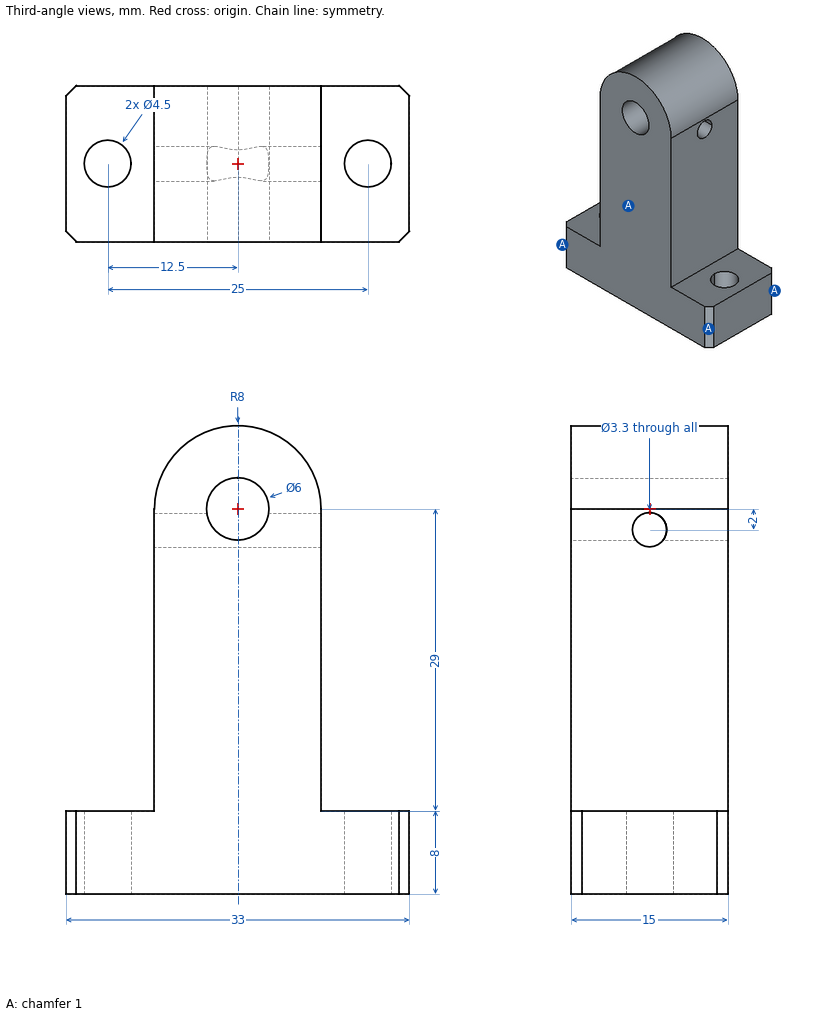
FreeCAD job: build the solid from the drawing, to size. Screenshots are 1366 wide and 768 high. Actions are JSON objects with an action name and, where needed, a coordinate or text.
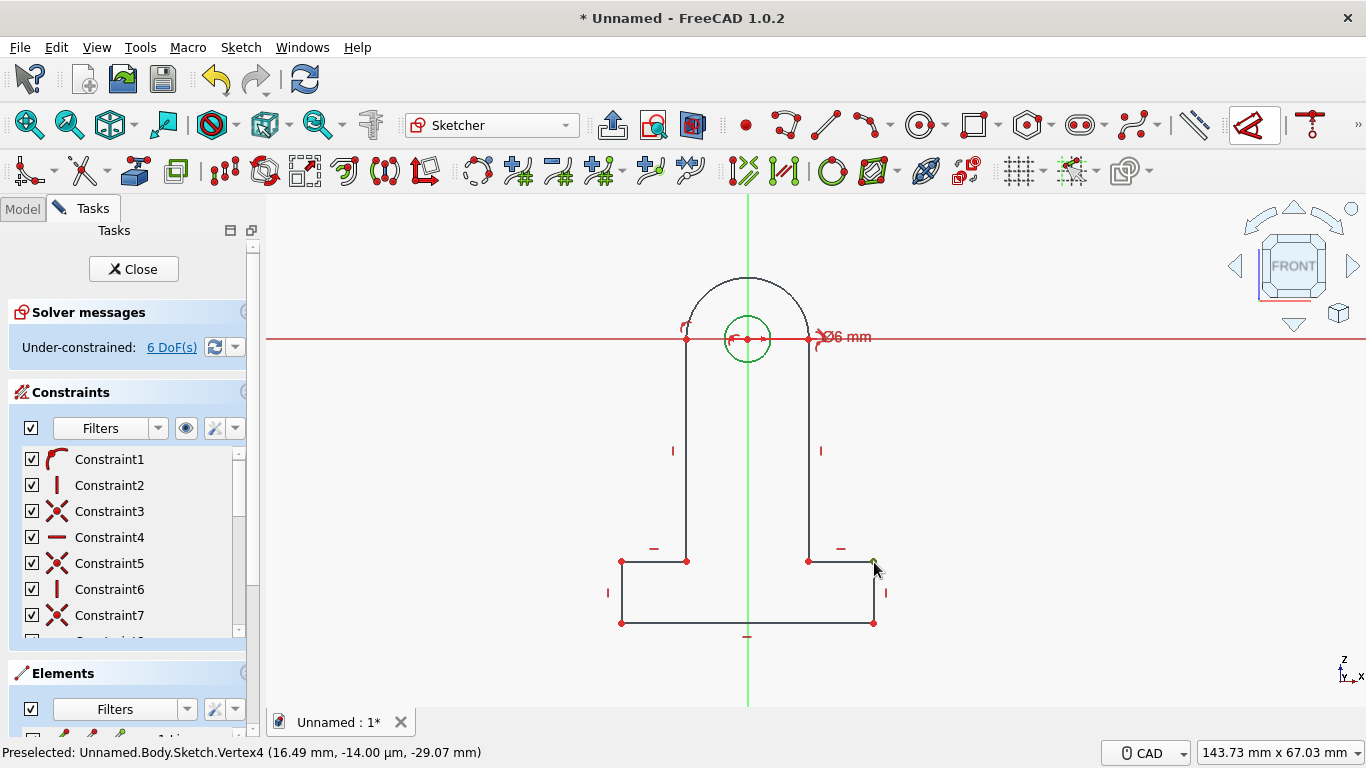
{"action": "left_click", "coordinate": [622, 562]}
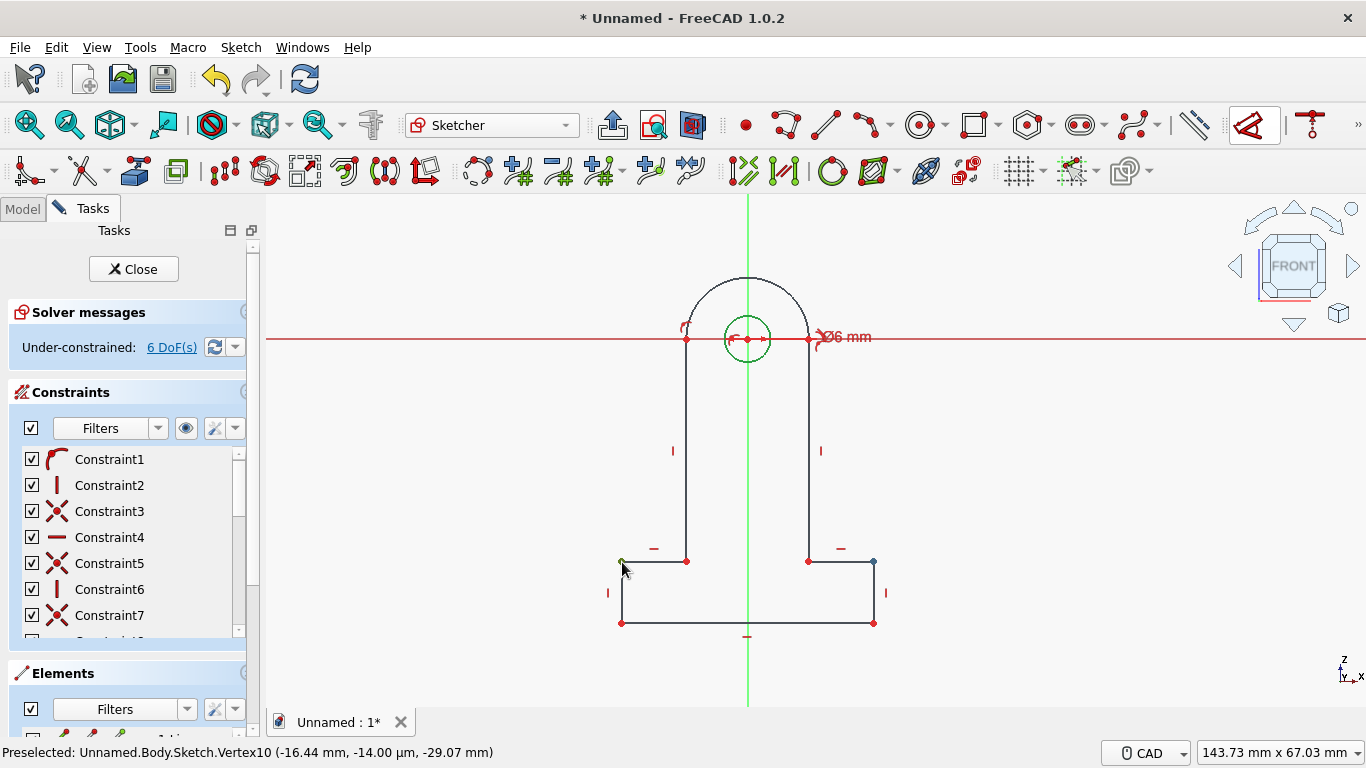
{"action": "left_click", "coordinate": [748, 581]}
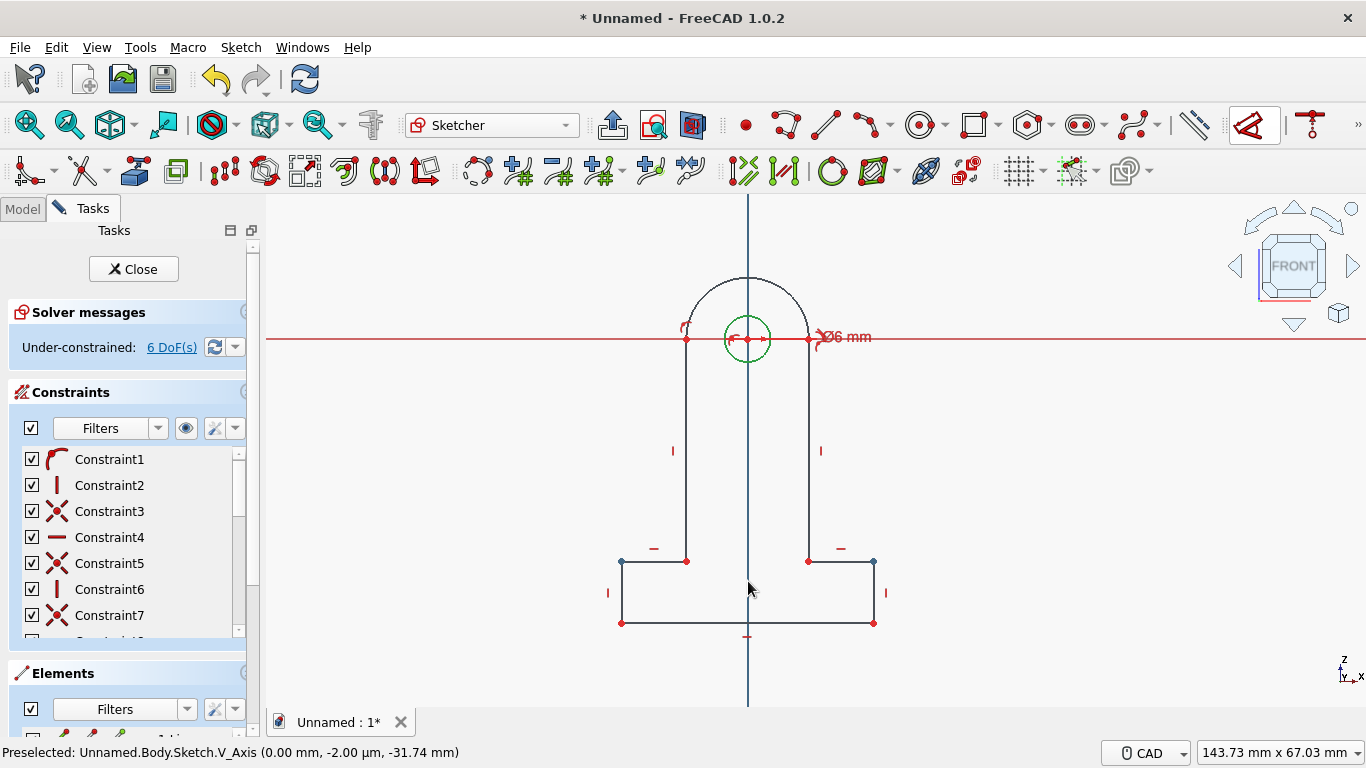
{"action": "key", "text": "s"}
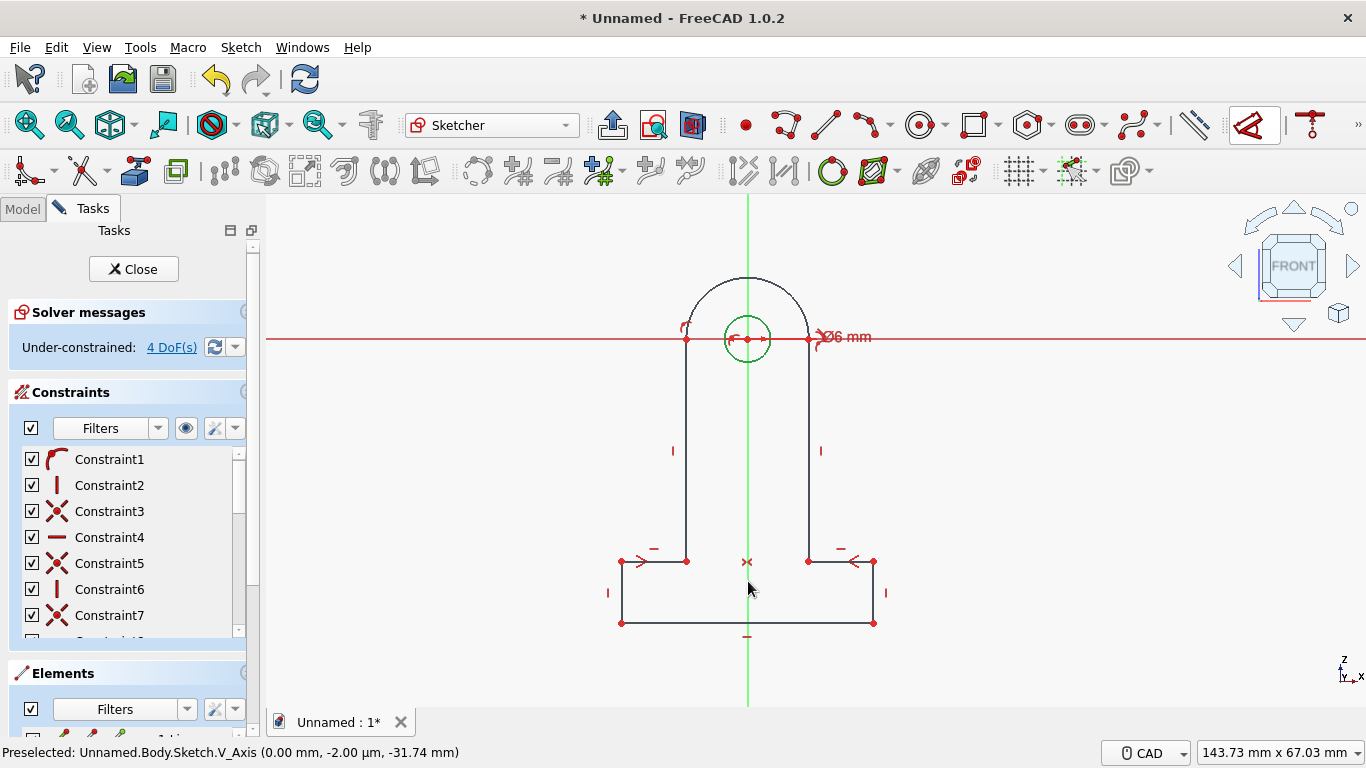
{"action": "key", "text": "d"}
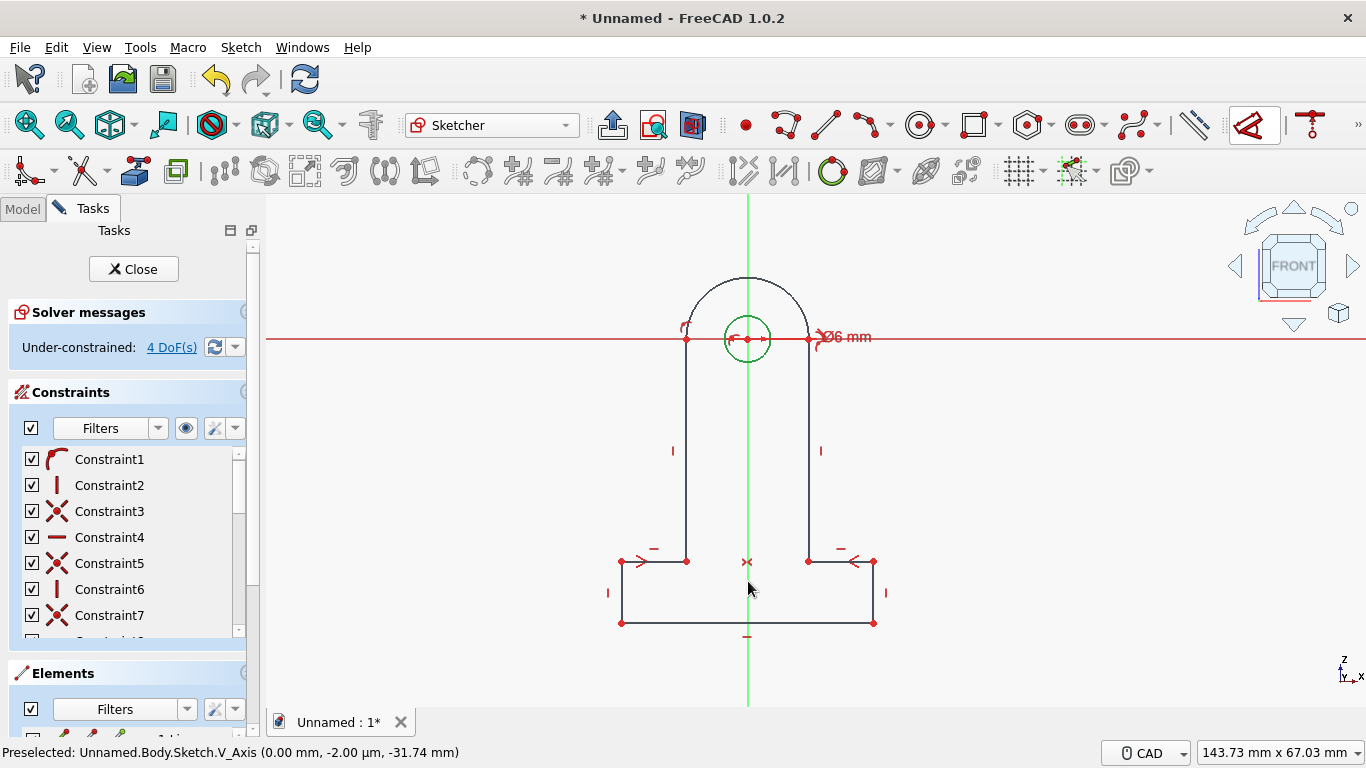
{"action": "left_click", "coordinate": [784, 290]}
{"action": "left_click", "coordinate": [803, 264]}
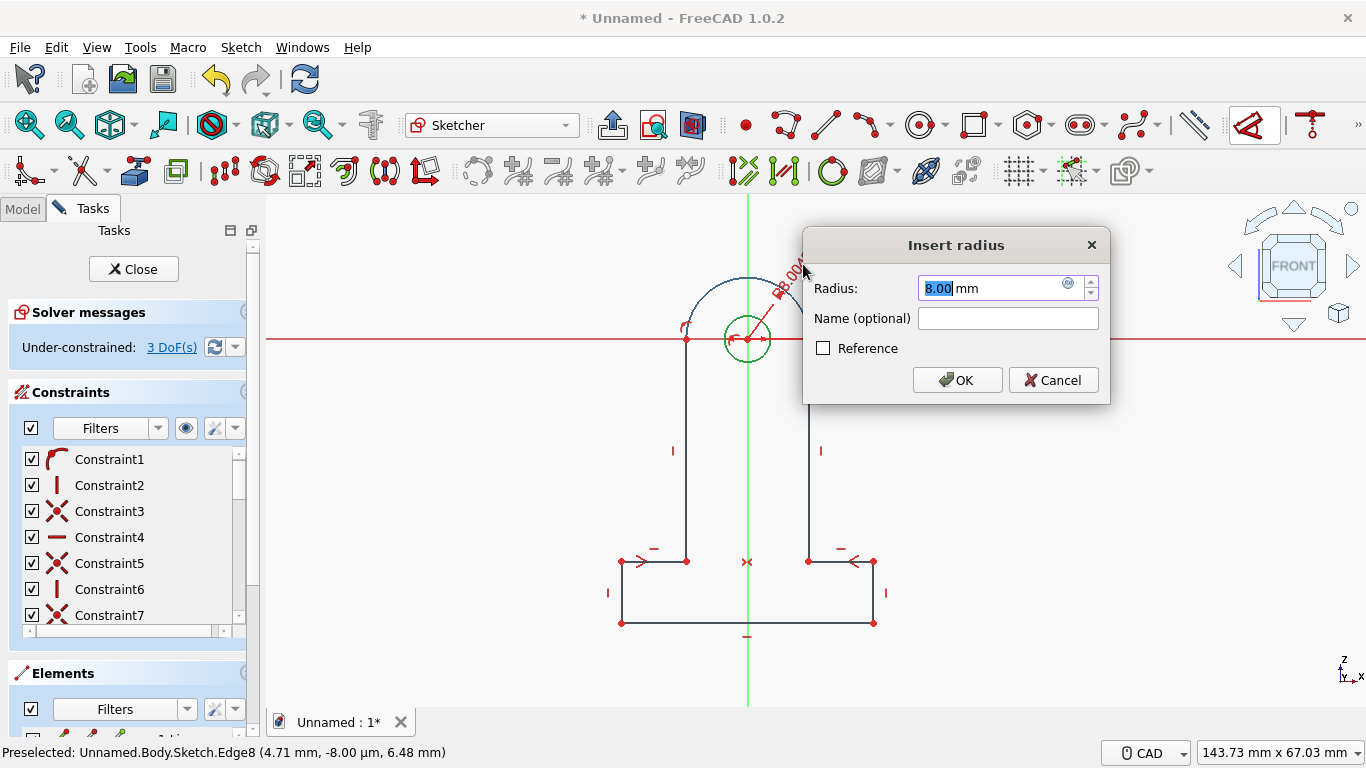
{"action": "type", "text": "8"}
{"action": "key", "text": "Return"}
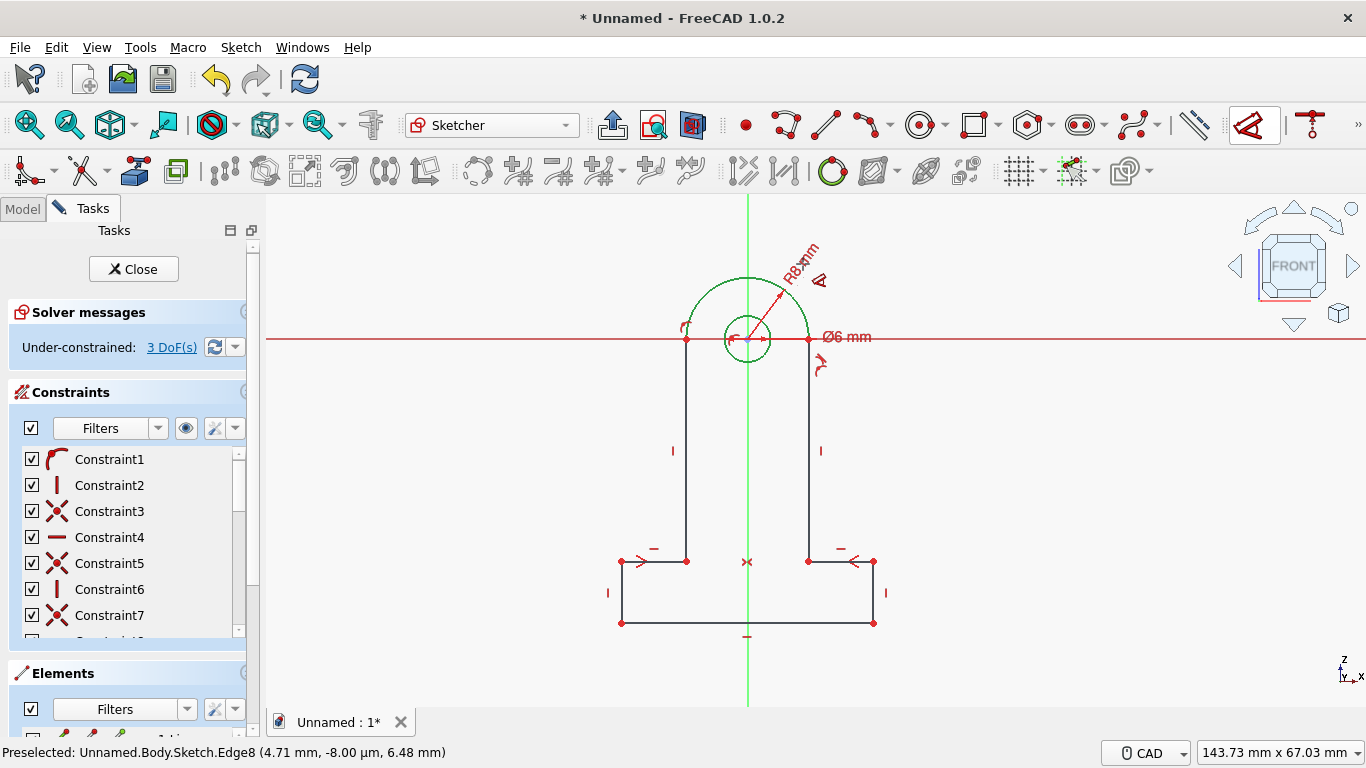
{"action": "left_click", "coordinate": [873, 580]}
{"action": "left_click", "coordinate": [907, 592]}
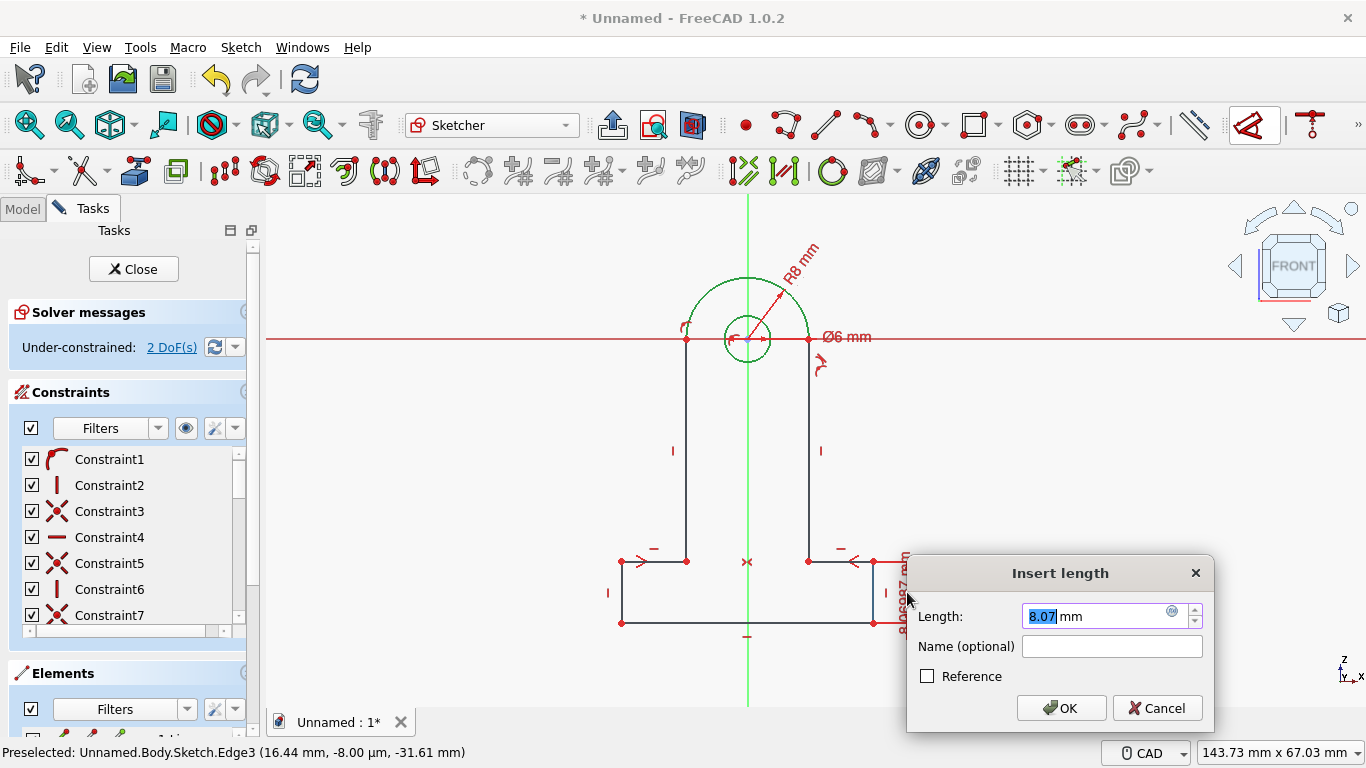
{"action": "type", "text": "8"}
{"action": "key", "text": "Return"}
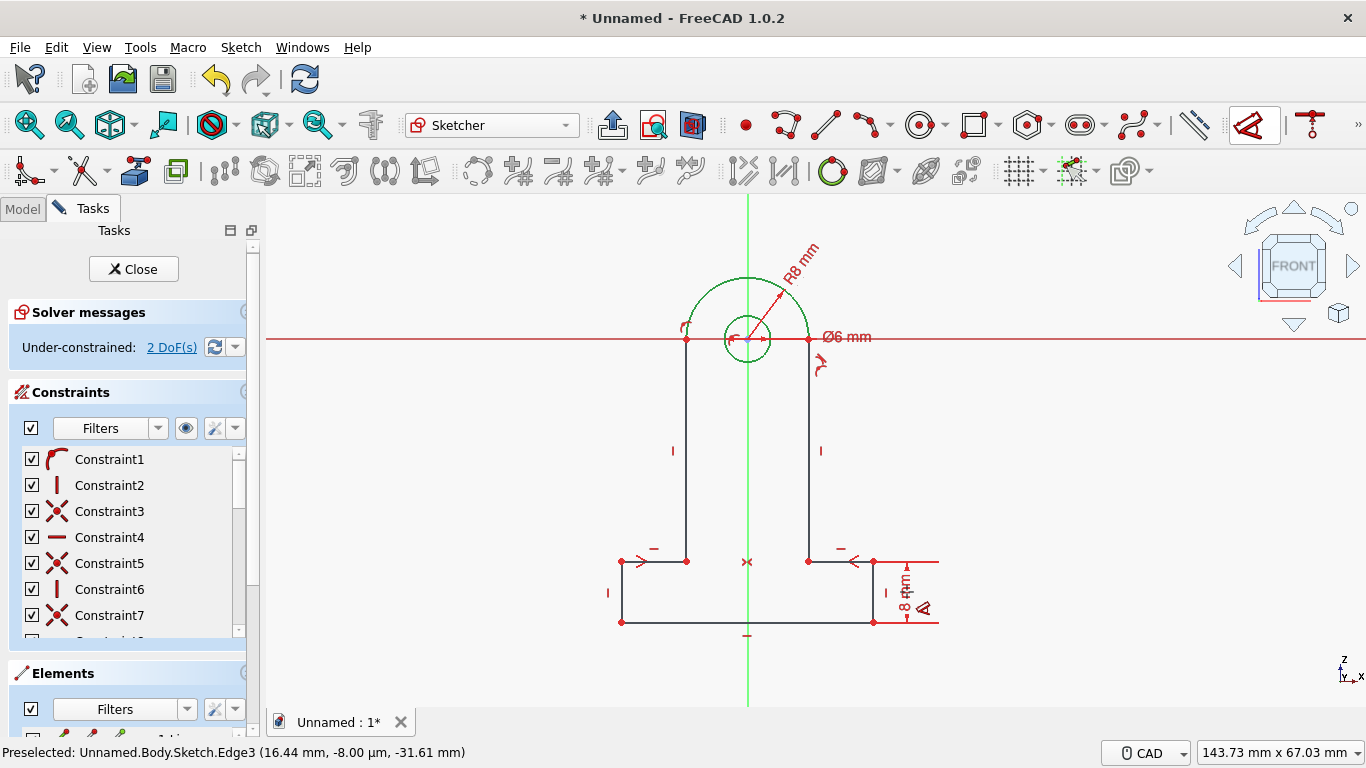
{"action": "left_click", "coordinate": [809, 406]}
{"action": "left_click", "coordinate": [843, 450]}